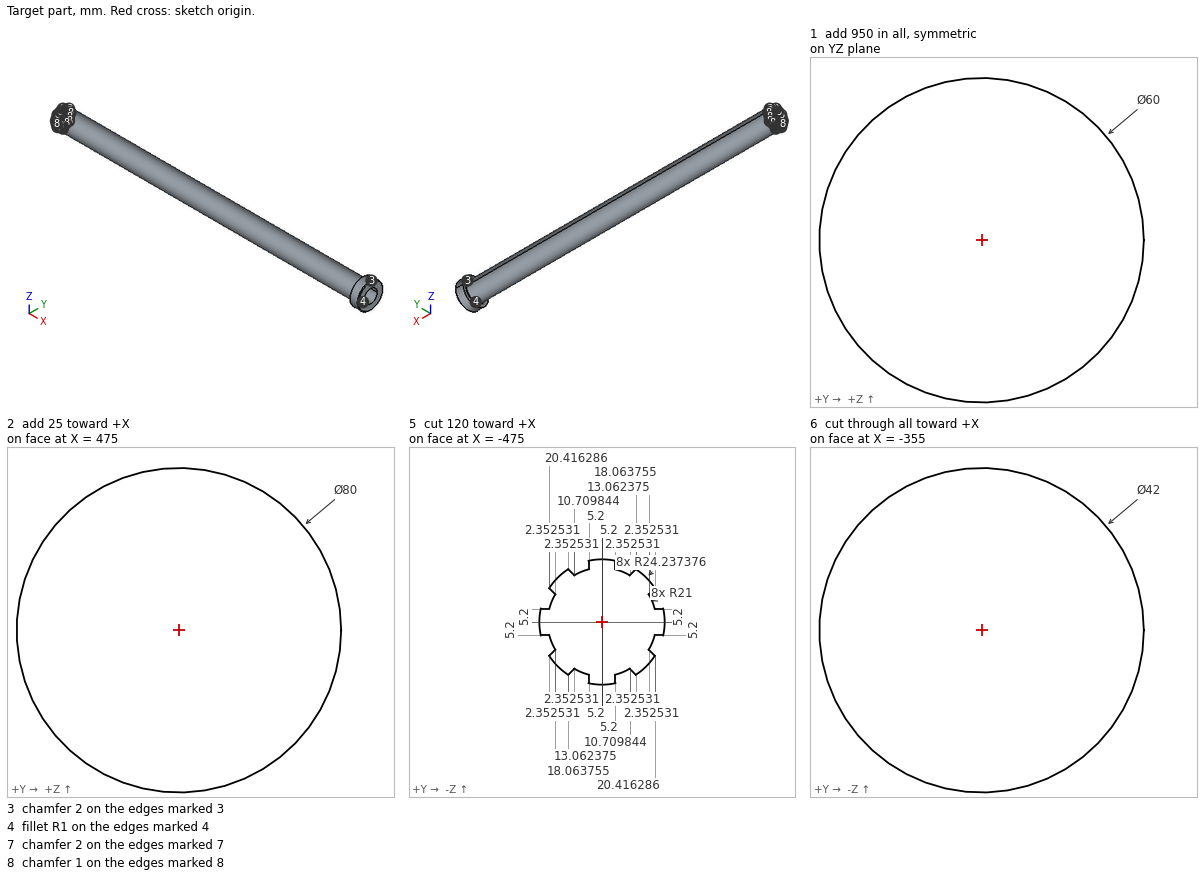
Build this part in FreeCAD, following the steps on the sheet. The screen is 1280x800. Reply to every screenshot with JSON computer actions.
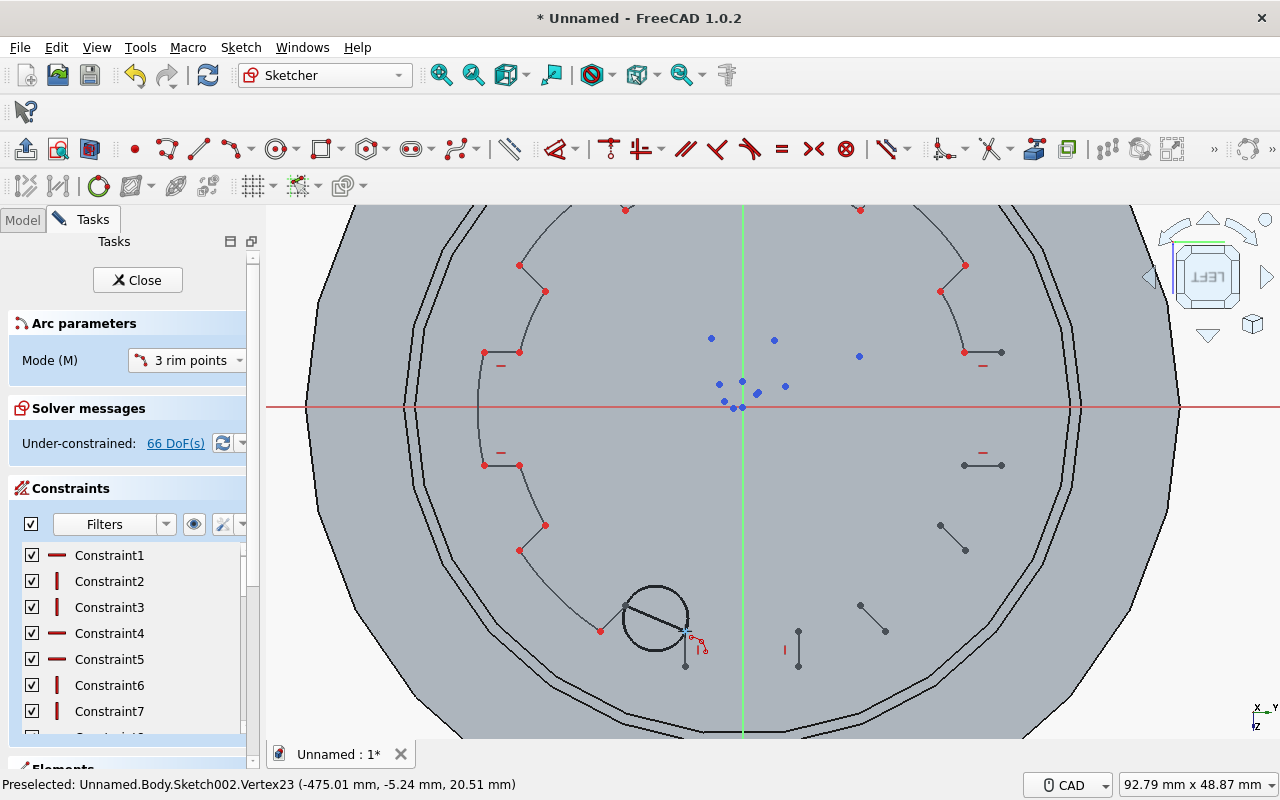
{"action": "scroll", "coordinate": [655, 619], "scroll_direction": "up", "scroll_amount": 10}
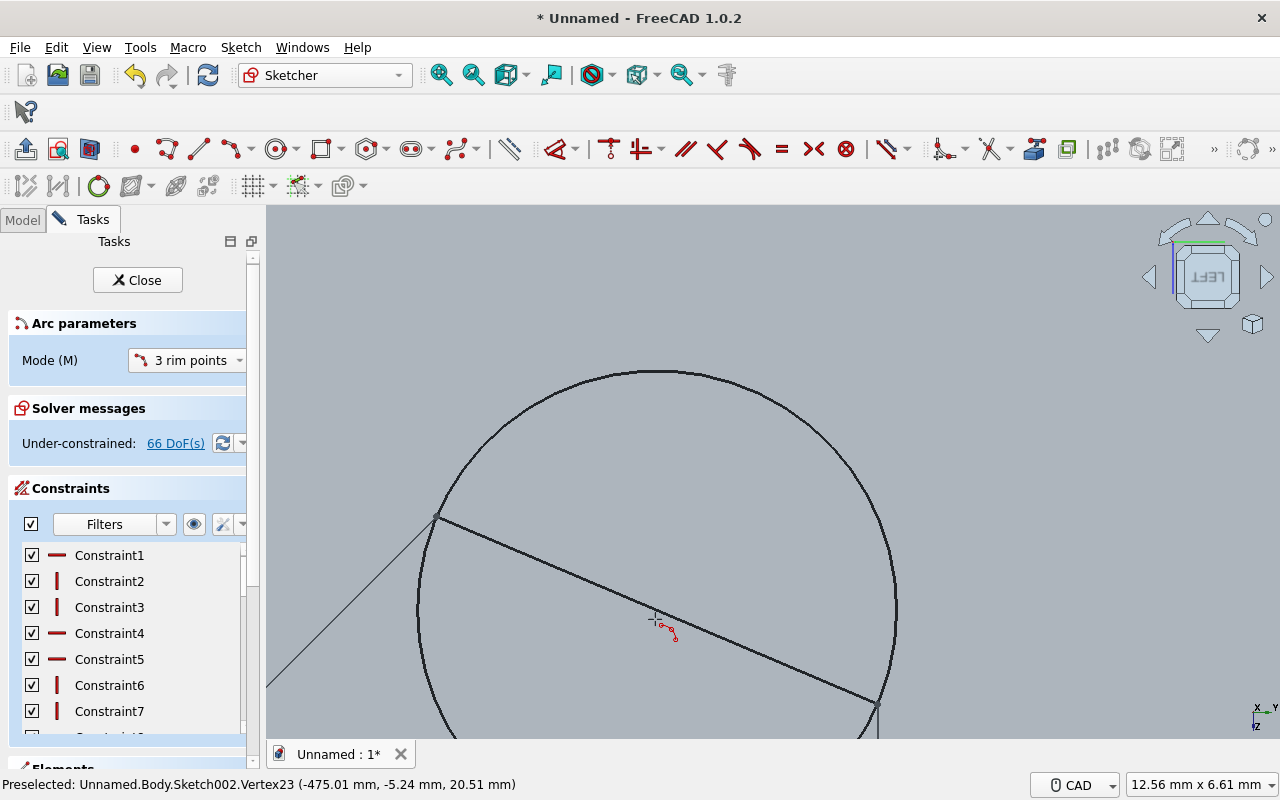
{"action": "left_click", "coordinate": [652, 615]}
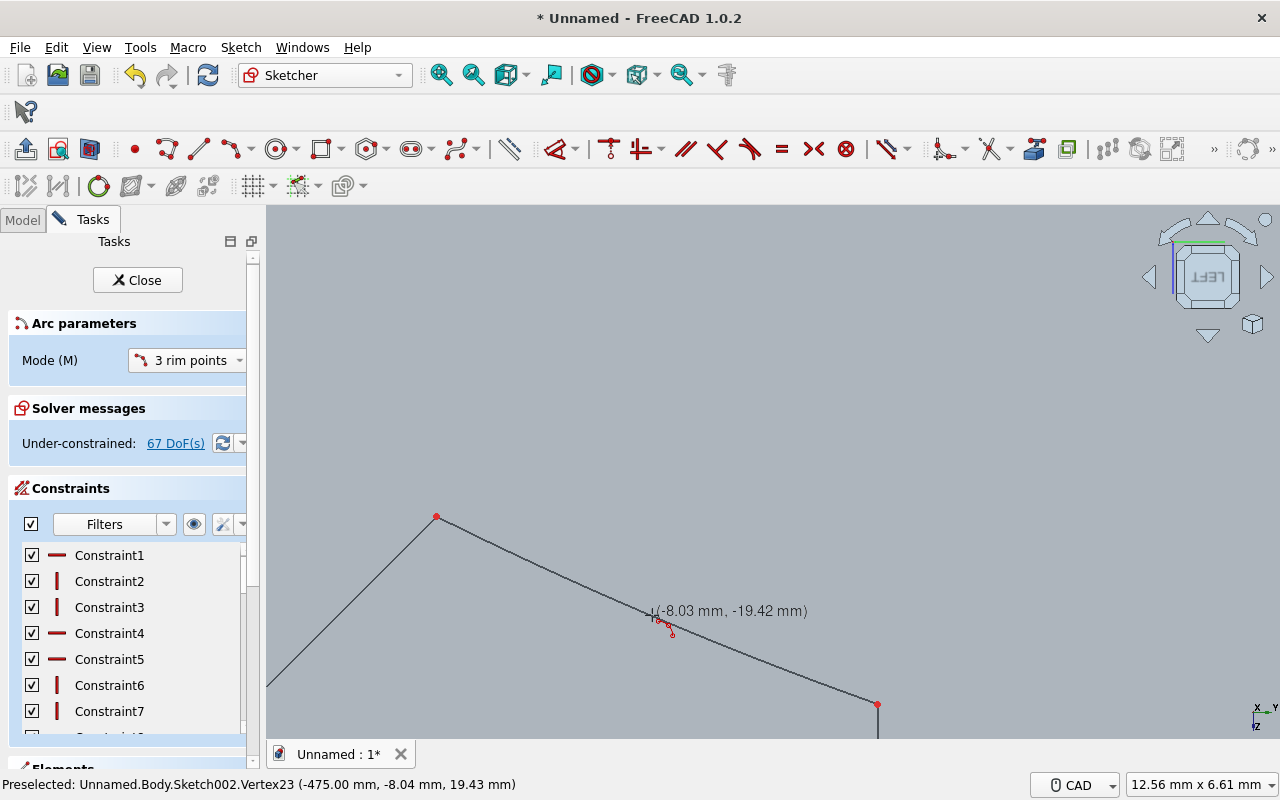
{"action": "scroll", "coordinate": [645, 614], "scroll_direction": "down", "scroll_amount": 12}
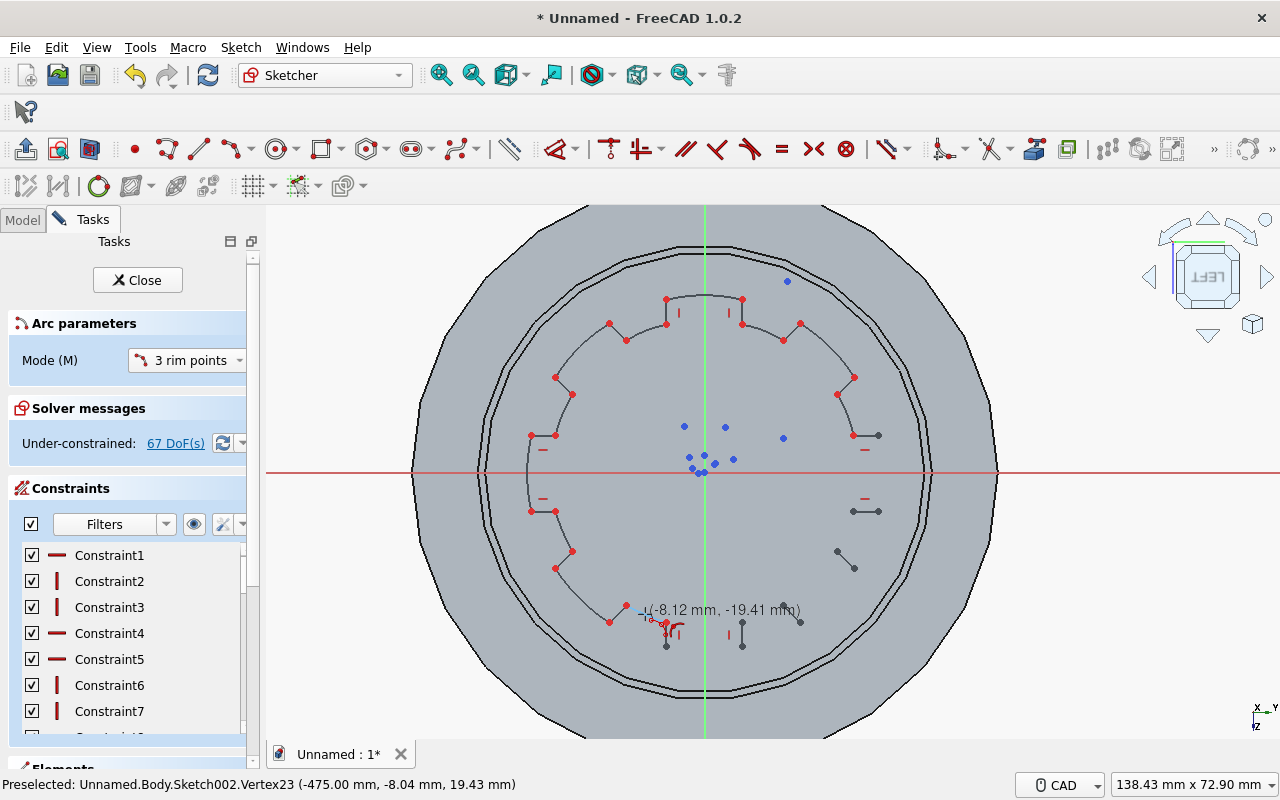
{"action": "scroll", "coordinate": [667, 646], "scroll_direction": "up", "scroll_amount": 2}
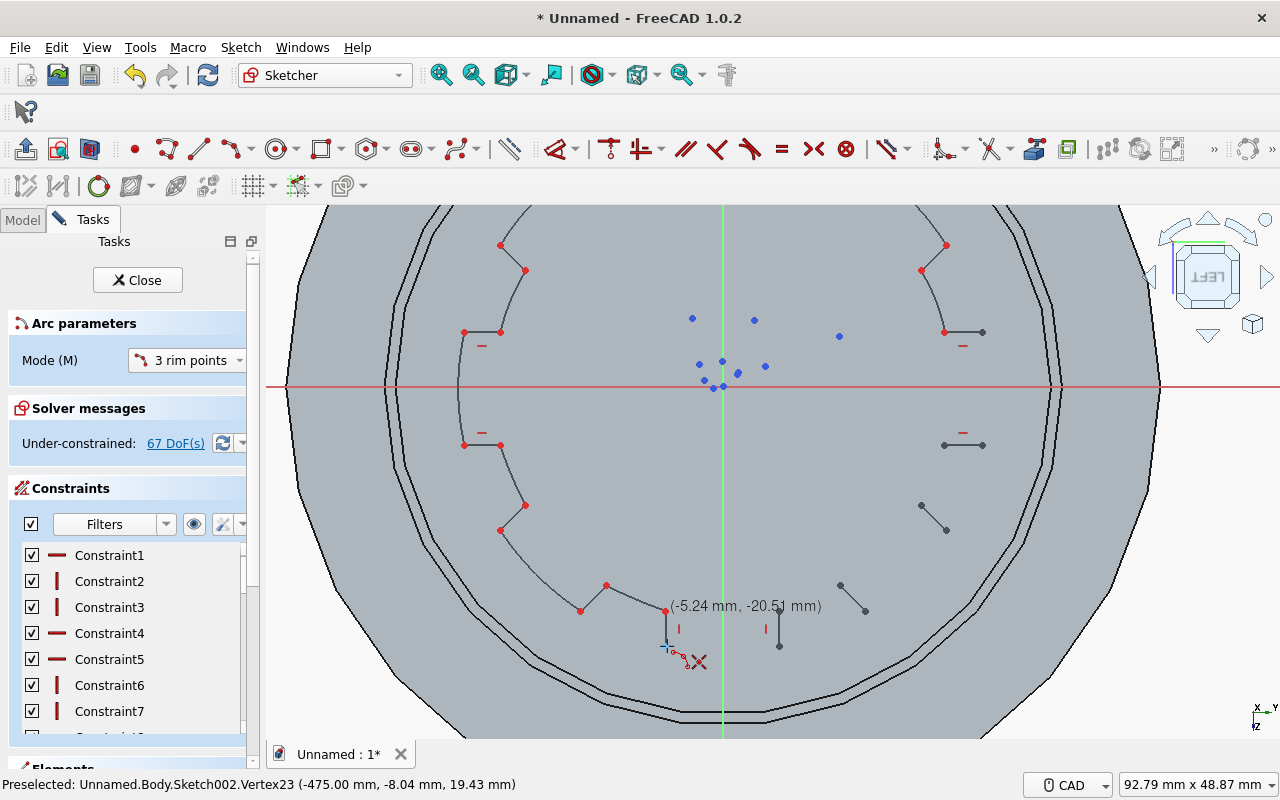
{"action": "left_click", "coordinate": [666, 647]}
{"action": "left_click", "coordinate": [779, 647]}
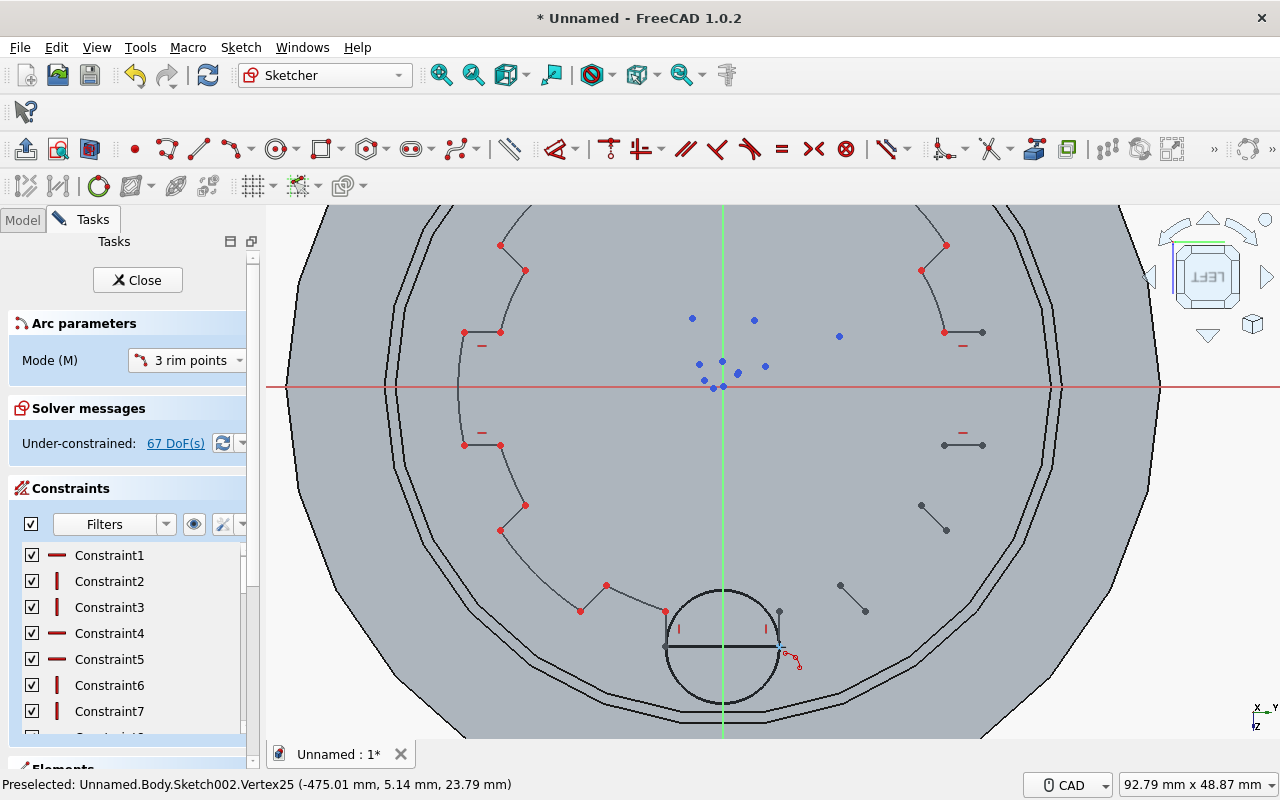
{"action": "scroll", "coordinate": [712, 652], "scroll_direction": "up", "scroll_amount": 5}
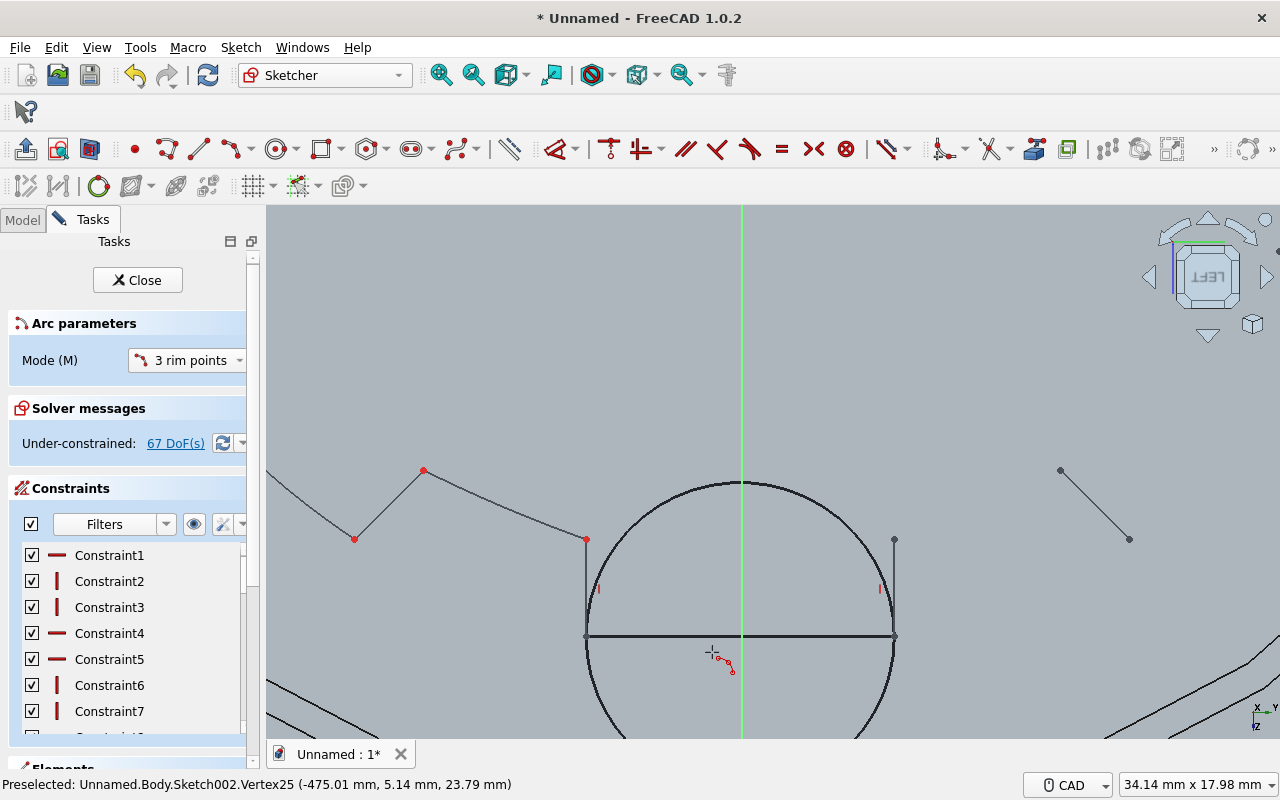
{"action": "left_click", "coordinate": [711, 649]}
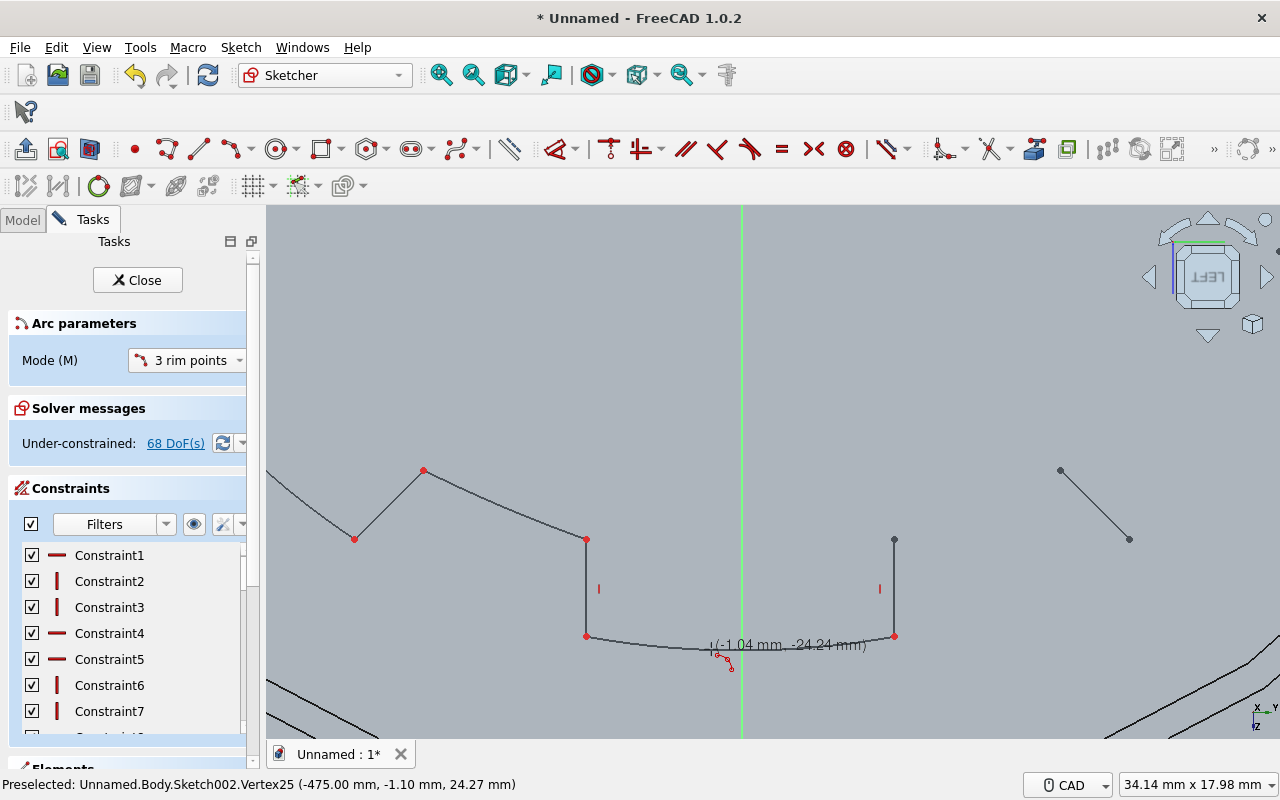
{"action": "scroll", "coordinate": [692, 649], "scroll_direction": "down", "scroll_amount": 7}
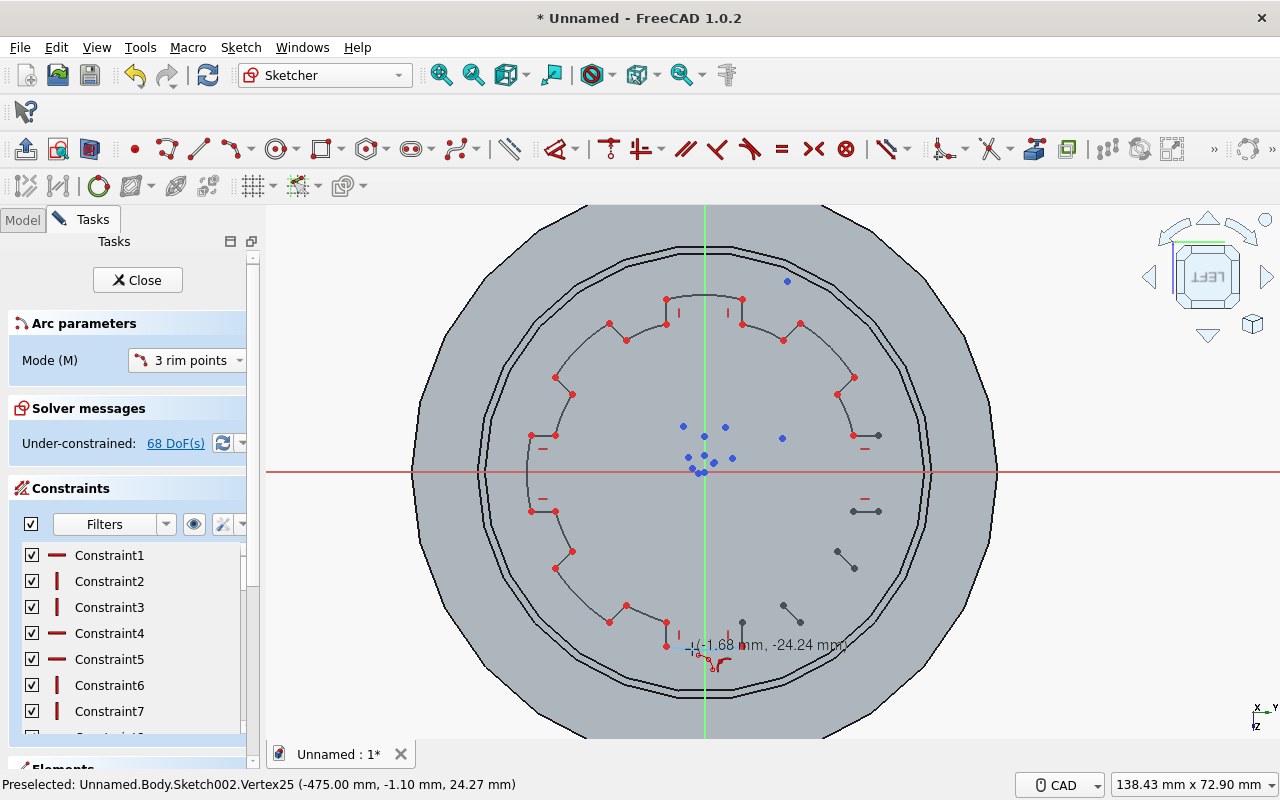
{"action": "scroll", "coordinate": [743, 621], "scroll_direction": "up", "scroll_amount": 2}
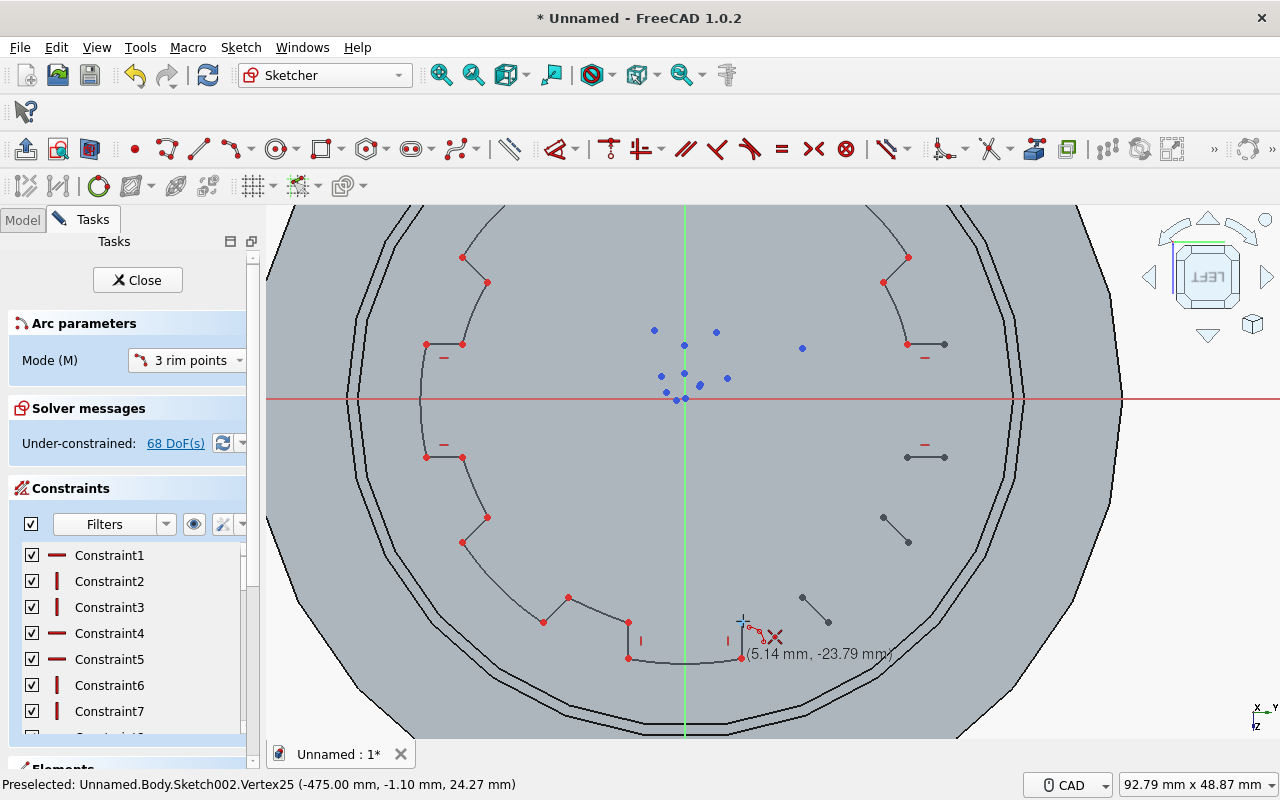
{"action": "left_click", "coordinate": [742, 623]}
{"action": "left_click", "coordinate": [803, 598]}